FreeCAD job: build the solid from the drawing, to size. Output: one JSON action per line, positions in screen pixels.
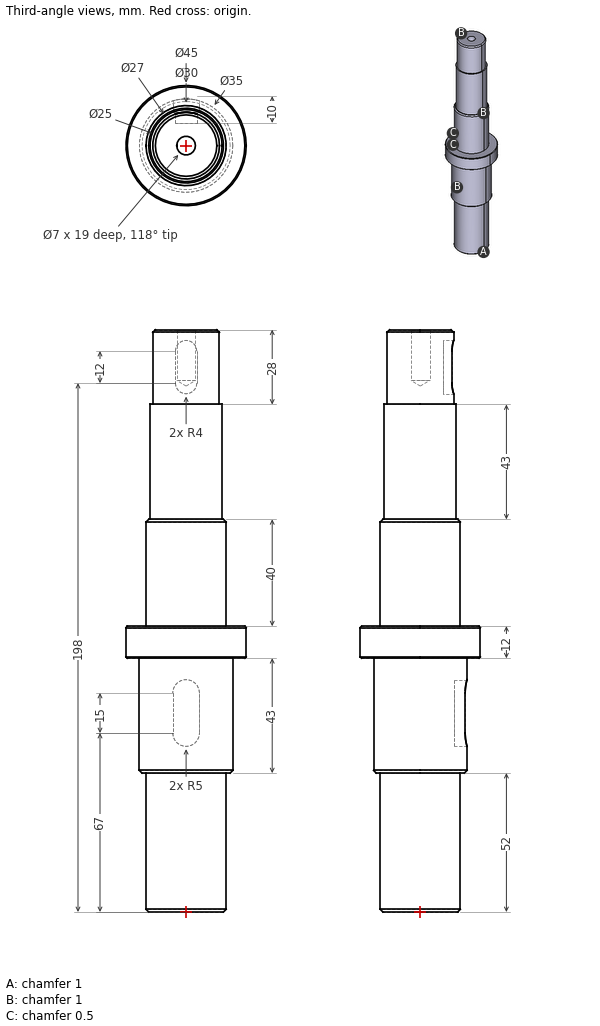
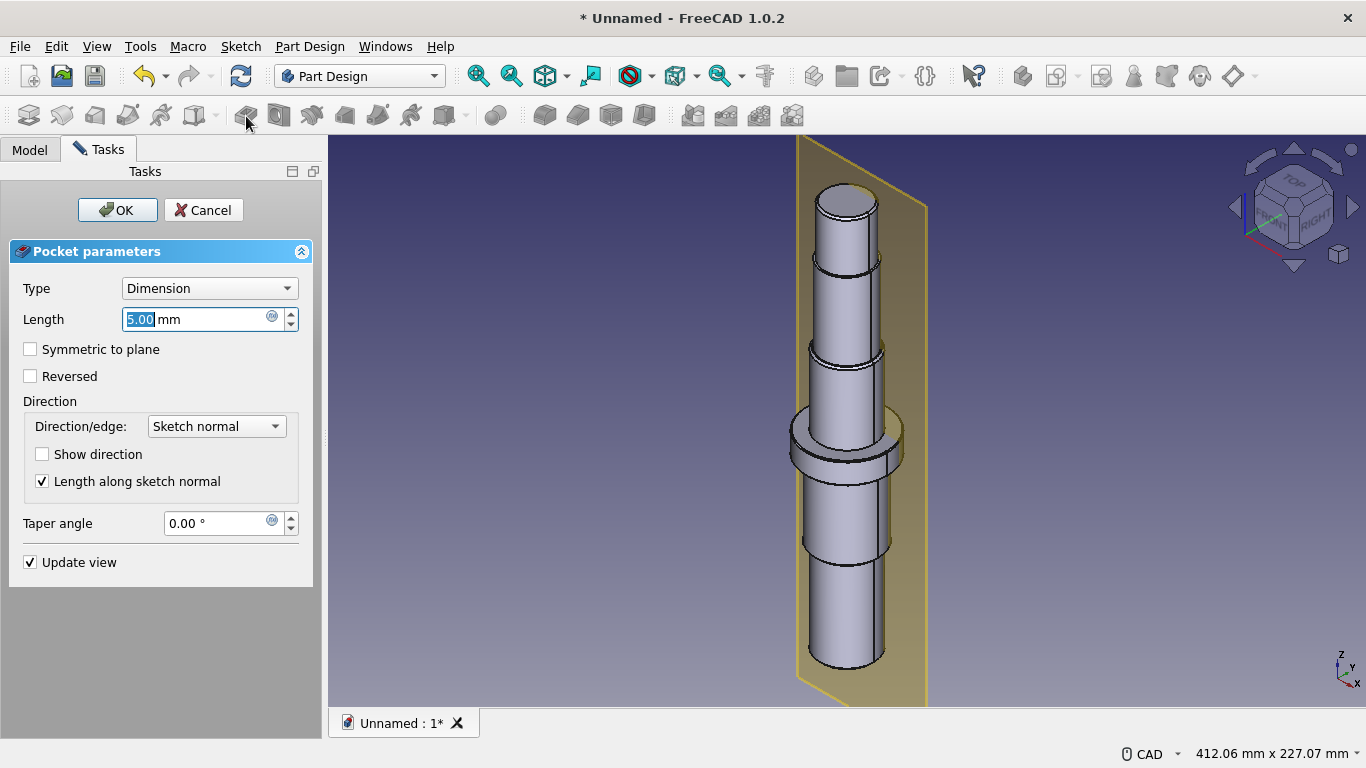
{"action": "type", "text": "10"}
{"action": "key", "text": "Tab"}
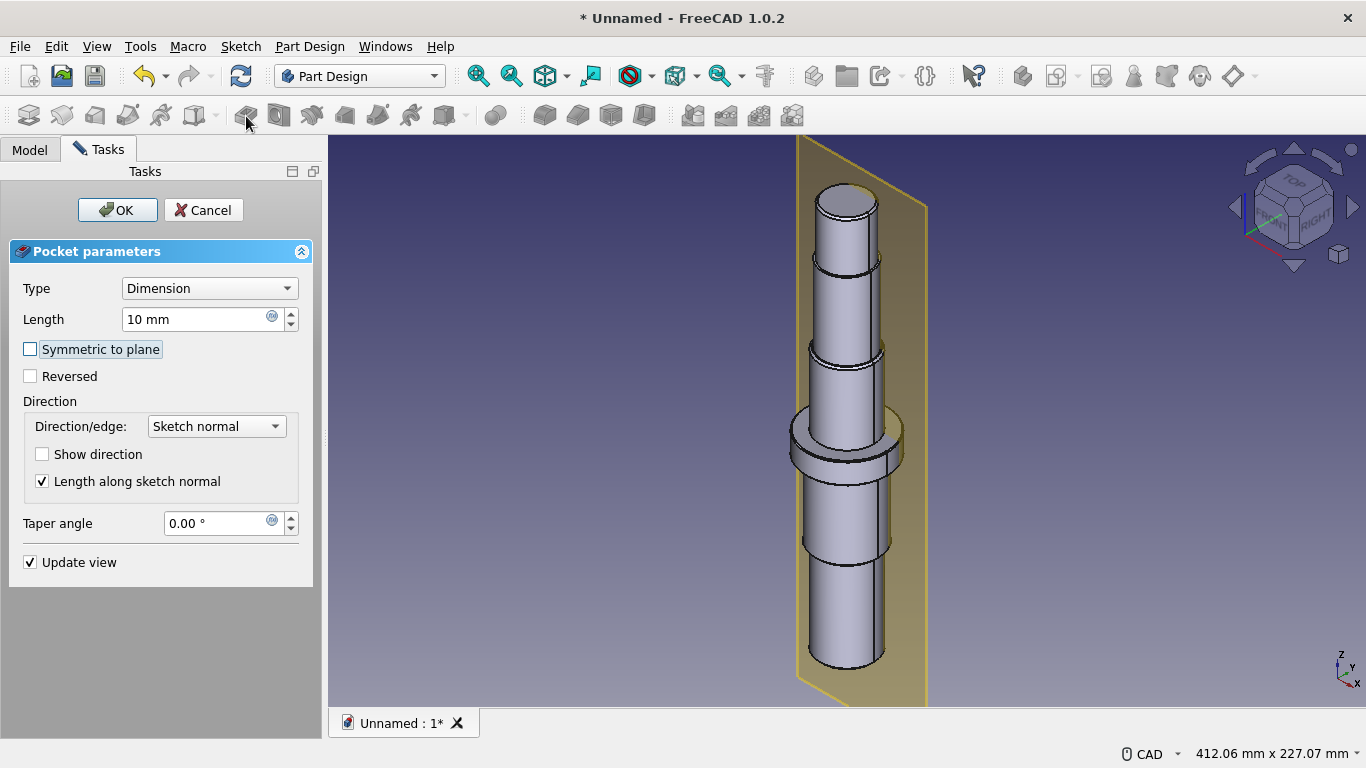
{"action": "left_click", "coordinate": [118, 210]}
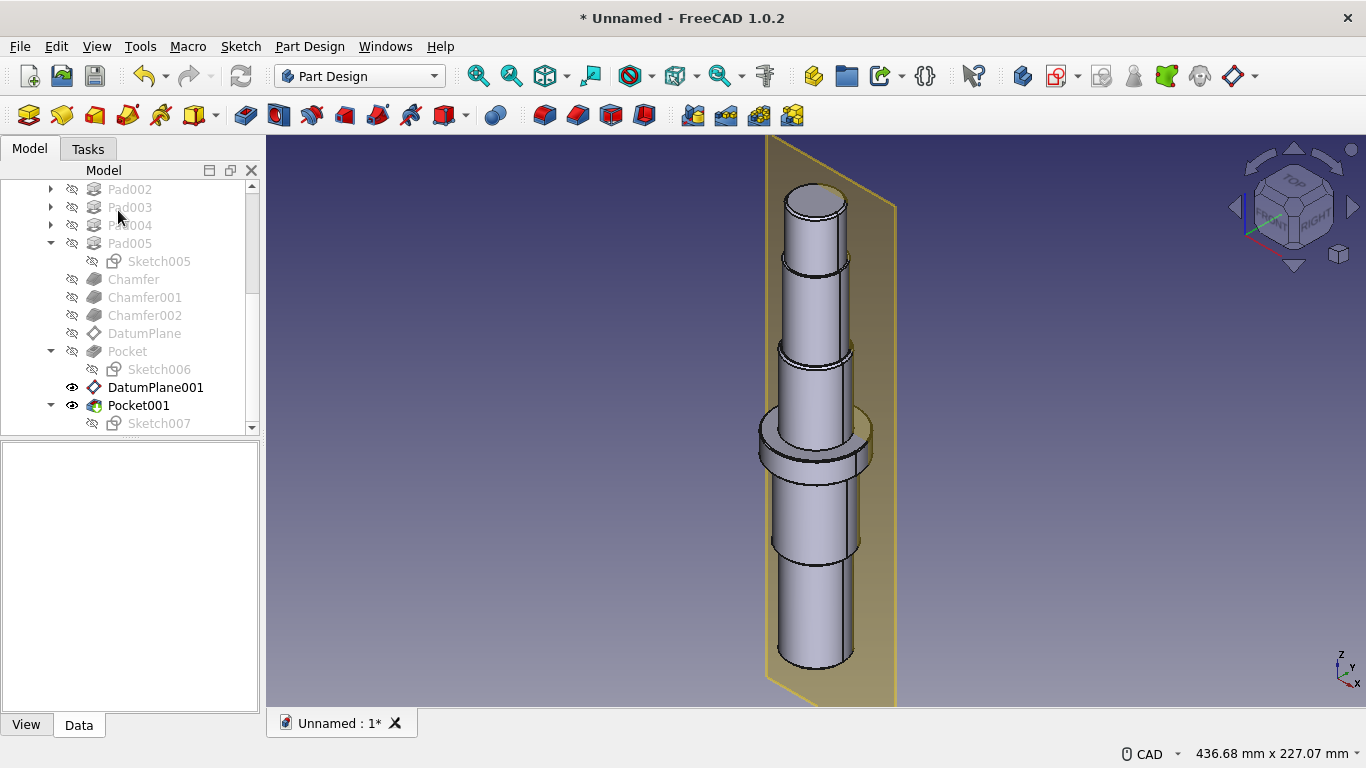
{"action": "left_click", "coordinate": [117, 387]}
{"action": "key", "text": "space"}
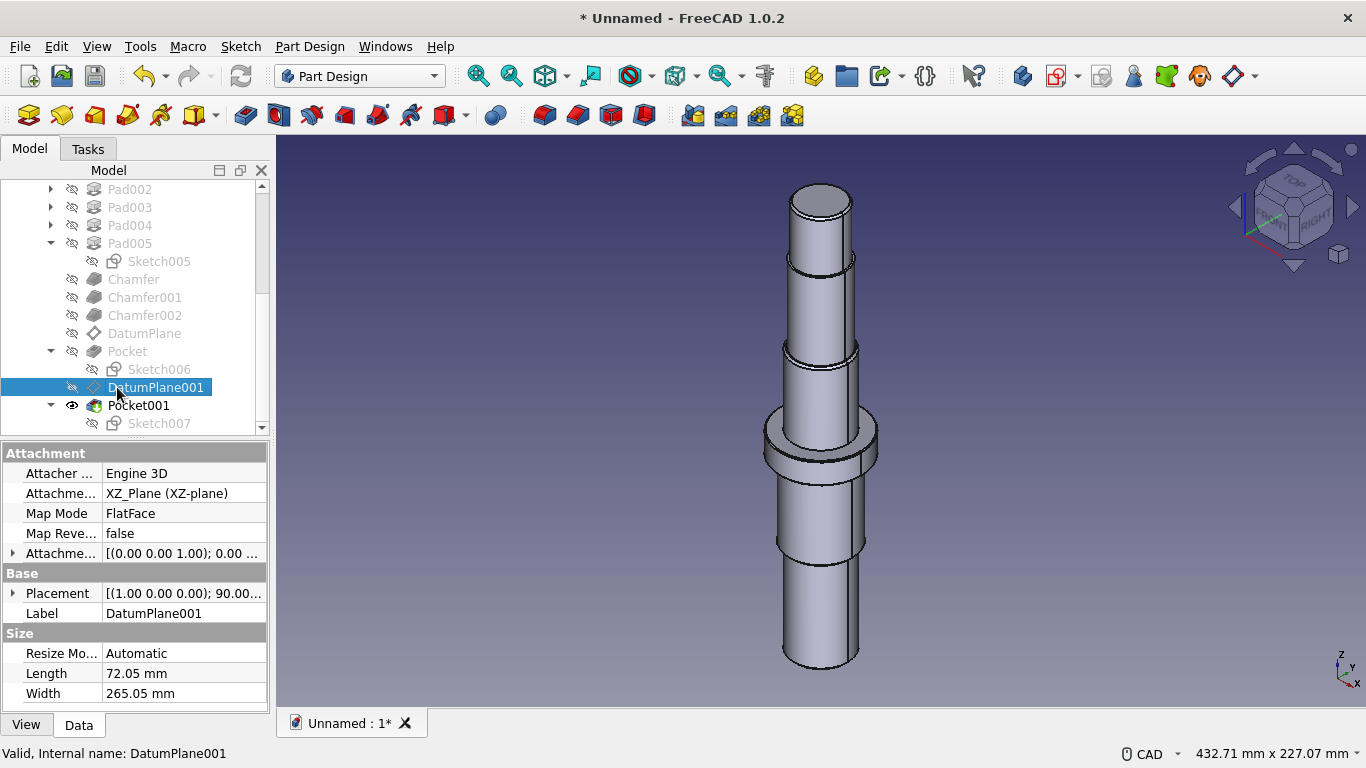
{"action": "left_click", "coordinate": [821, 200]}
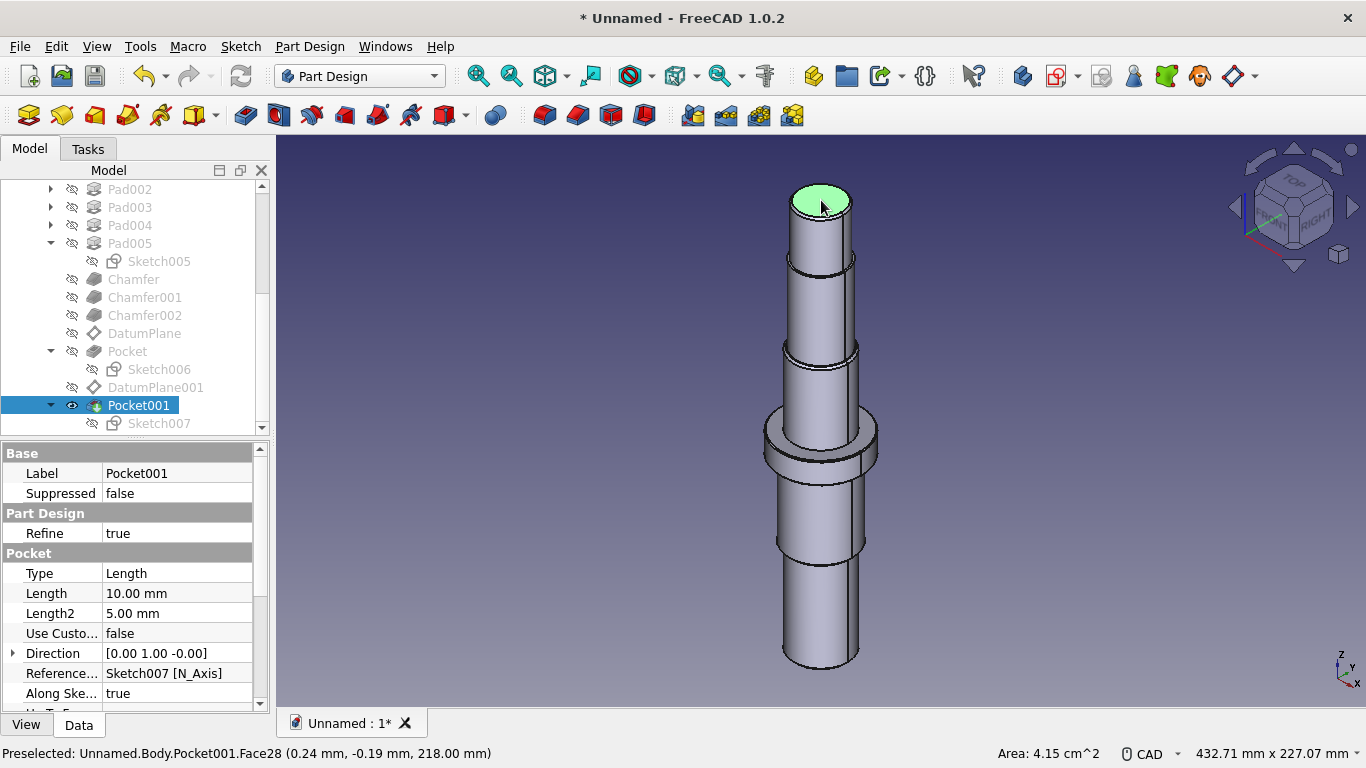
{"action": "left_click", "coordinate": [1056, 76]}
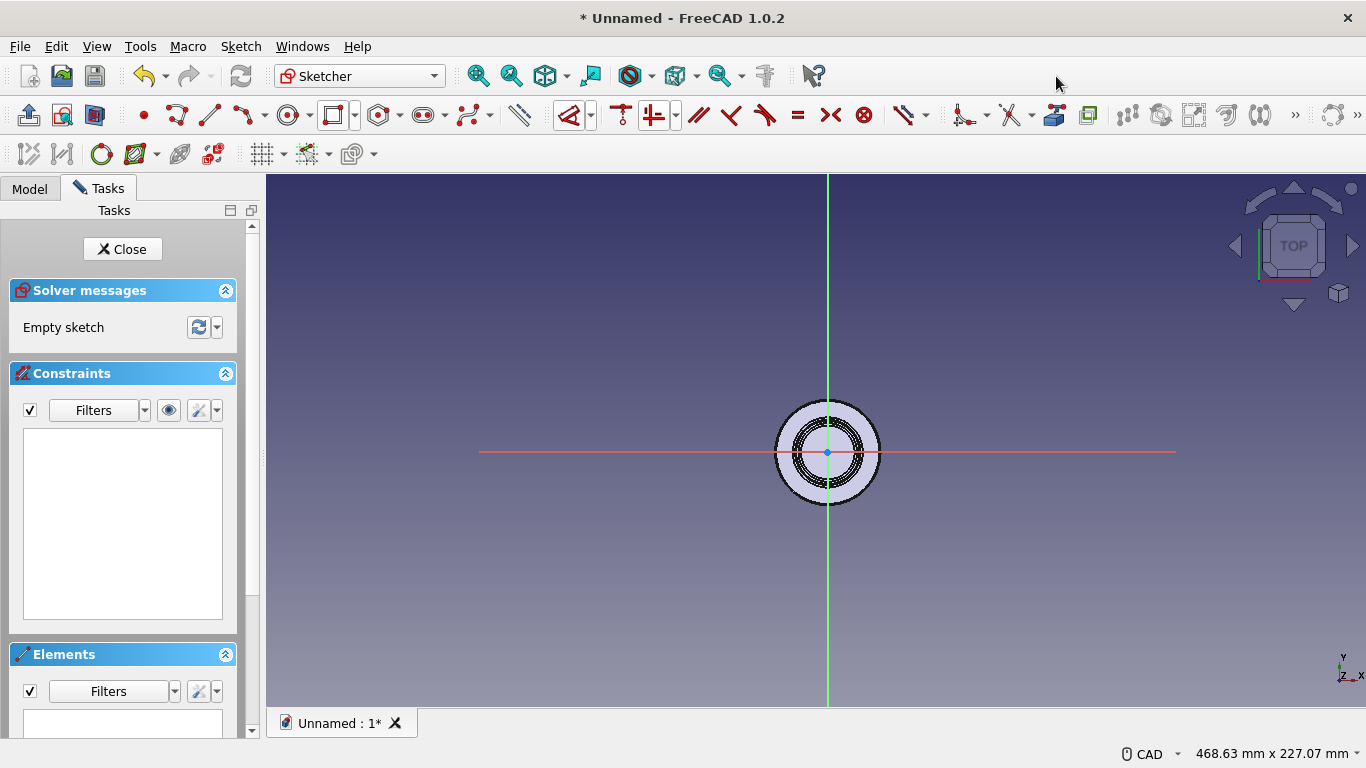
{"action": "scroll", "coordinate": [832, 453], "scroll_direction": "up", "scroll_amount": 15}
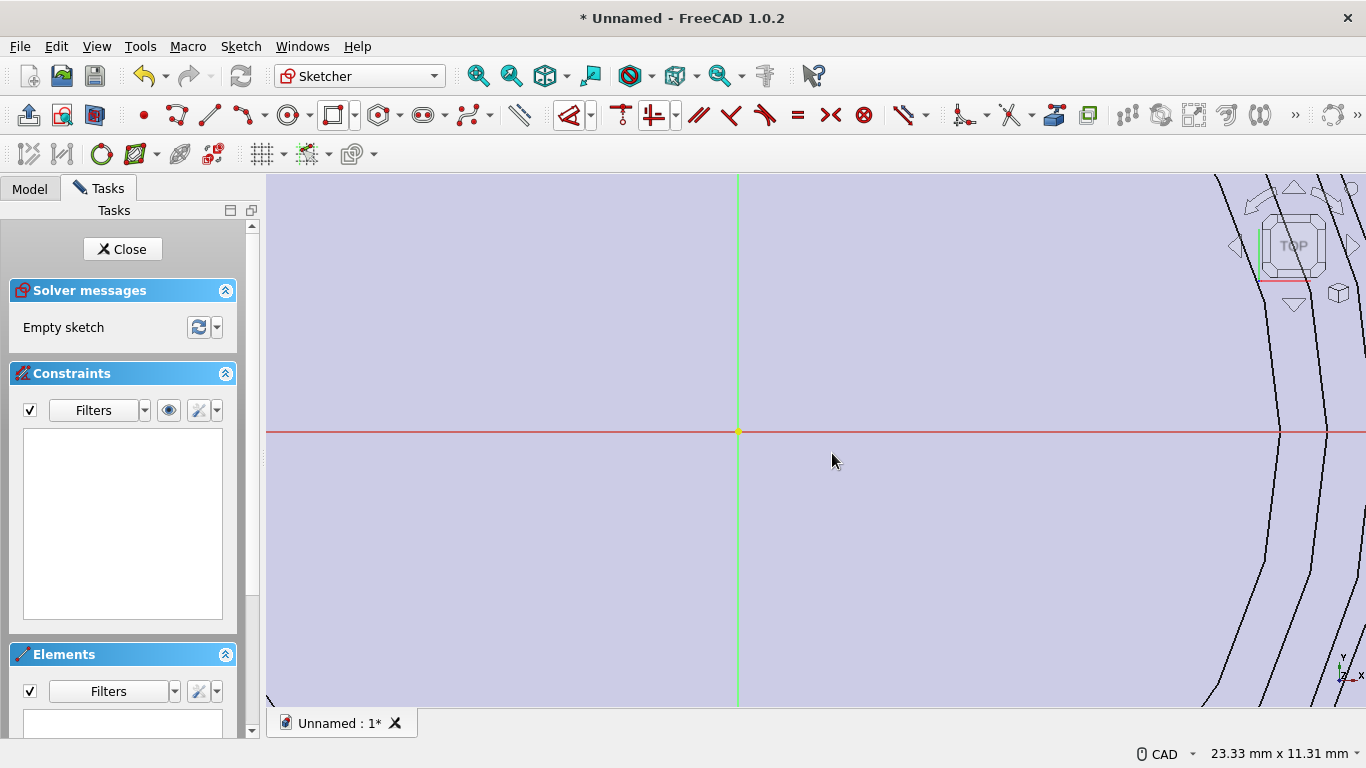
{"action": "key", "text": "g c"}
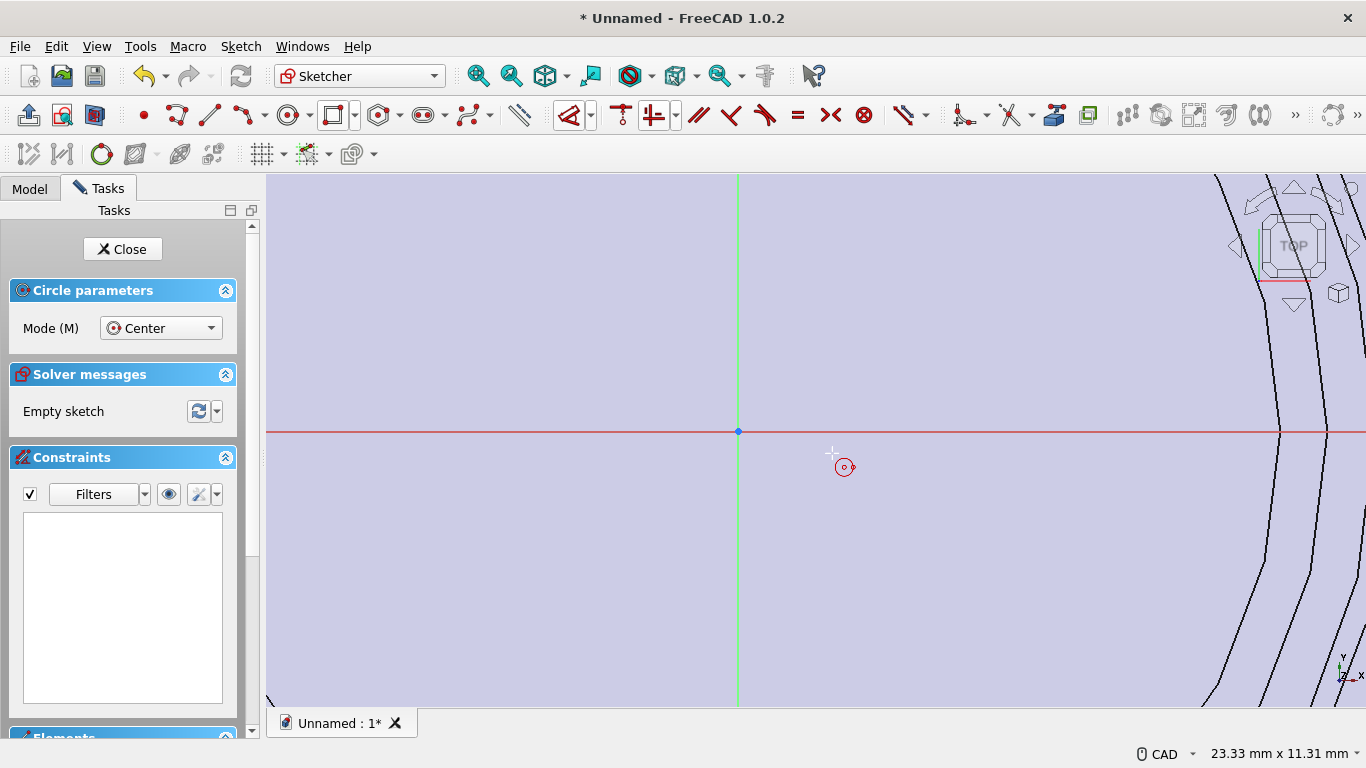
{"action": "left_click", "coordinate": [738, 432]}
{"action": "mouse_move", "coordinate": [855, 315]}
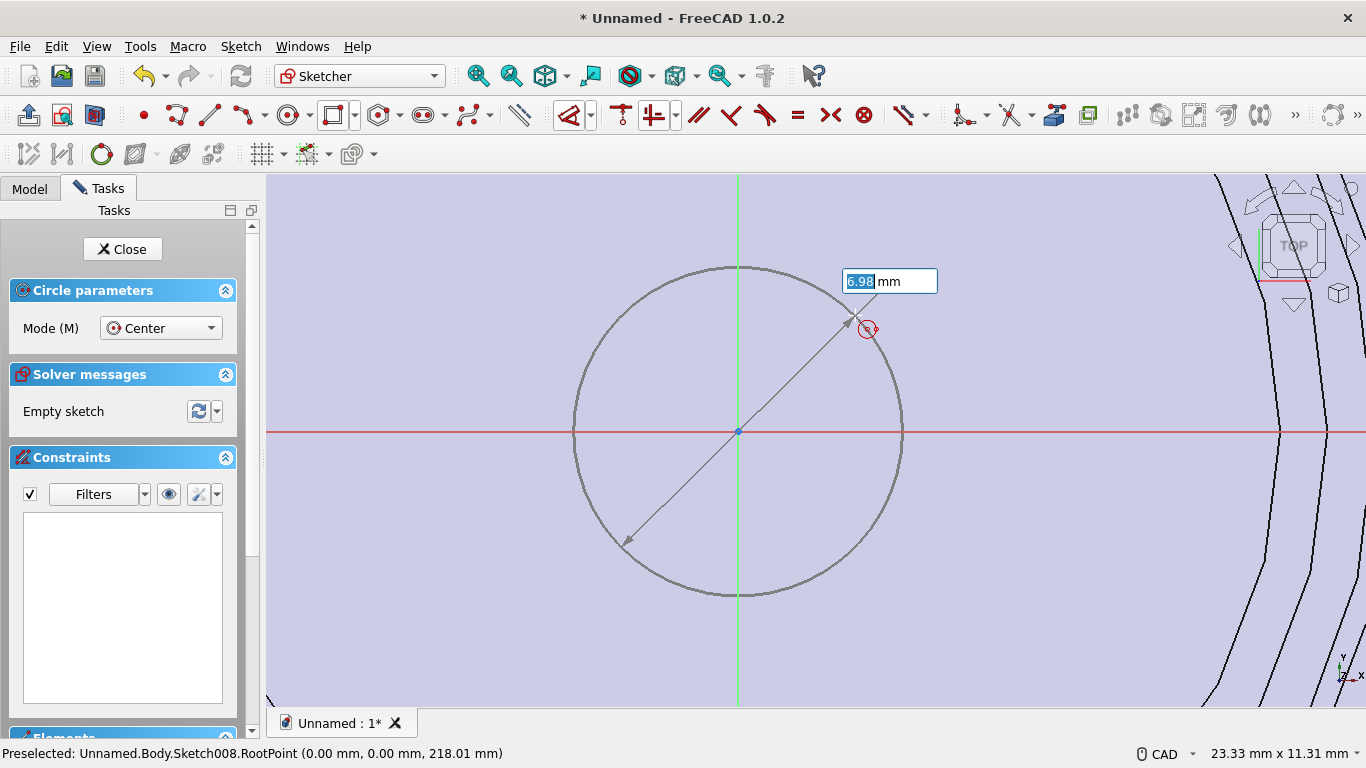
{"action": "type", "text": "7"}
{"action": "key", "text": "Return"}
{"action": "key", "text": "Escape"}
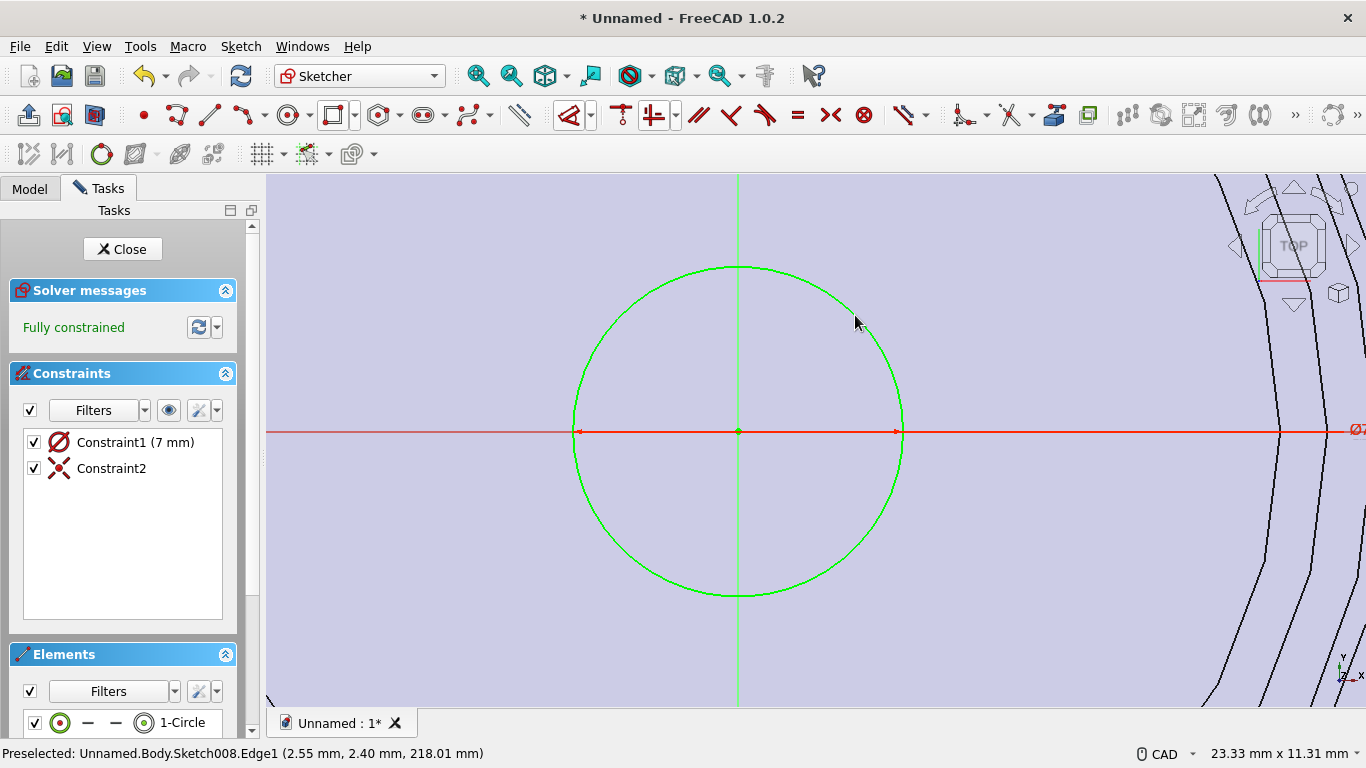
{"action": "left_click", "coordinate": [123, 249]}